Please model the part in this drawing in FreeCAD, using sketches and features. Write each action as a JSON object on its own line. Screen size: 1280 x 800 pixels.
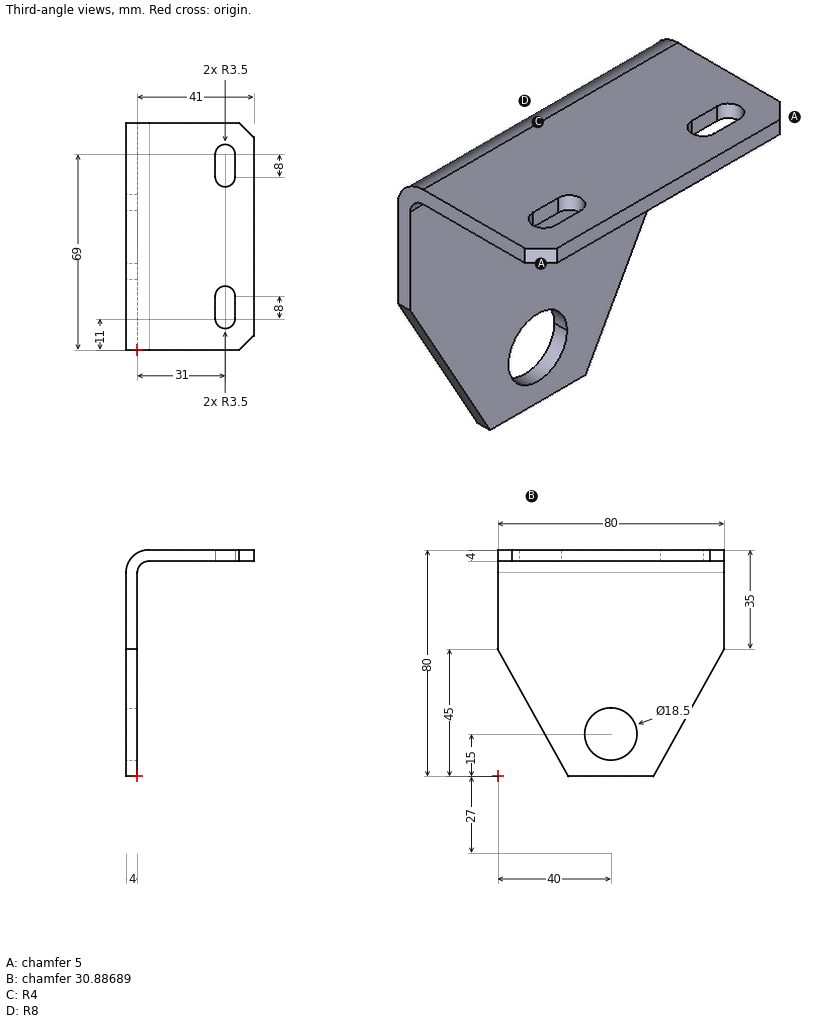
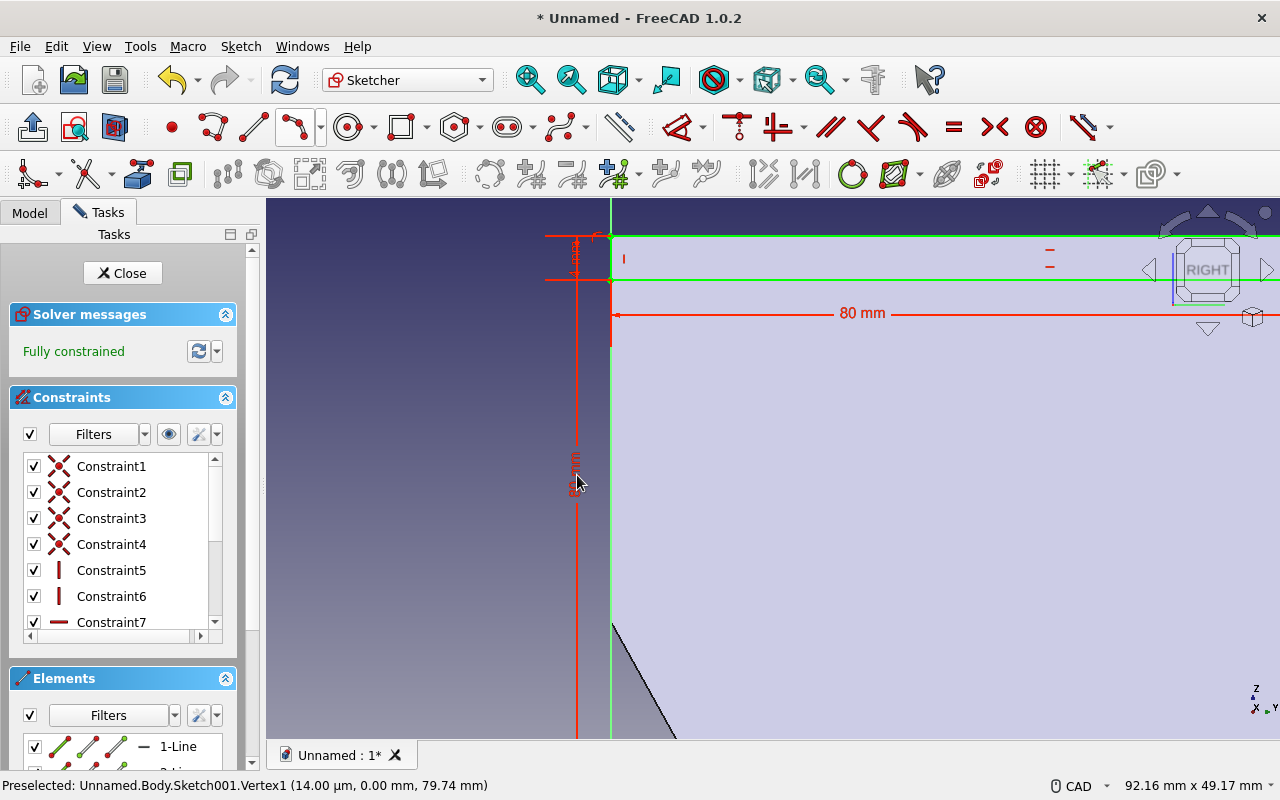
{"action": "left_click", "coordinate": [123, 273]}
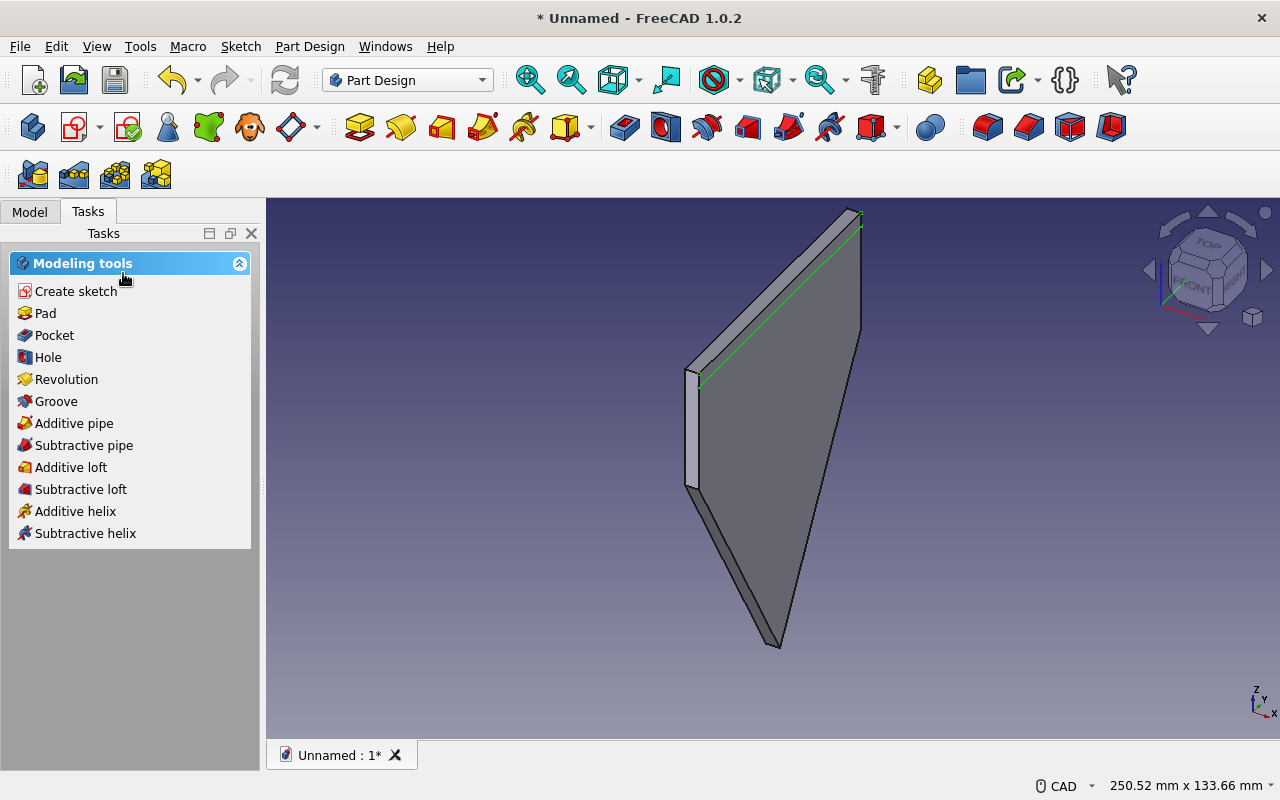
{"action": "left_click", "coordinate": [360, 128]}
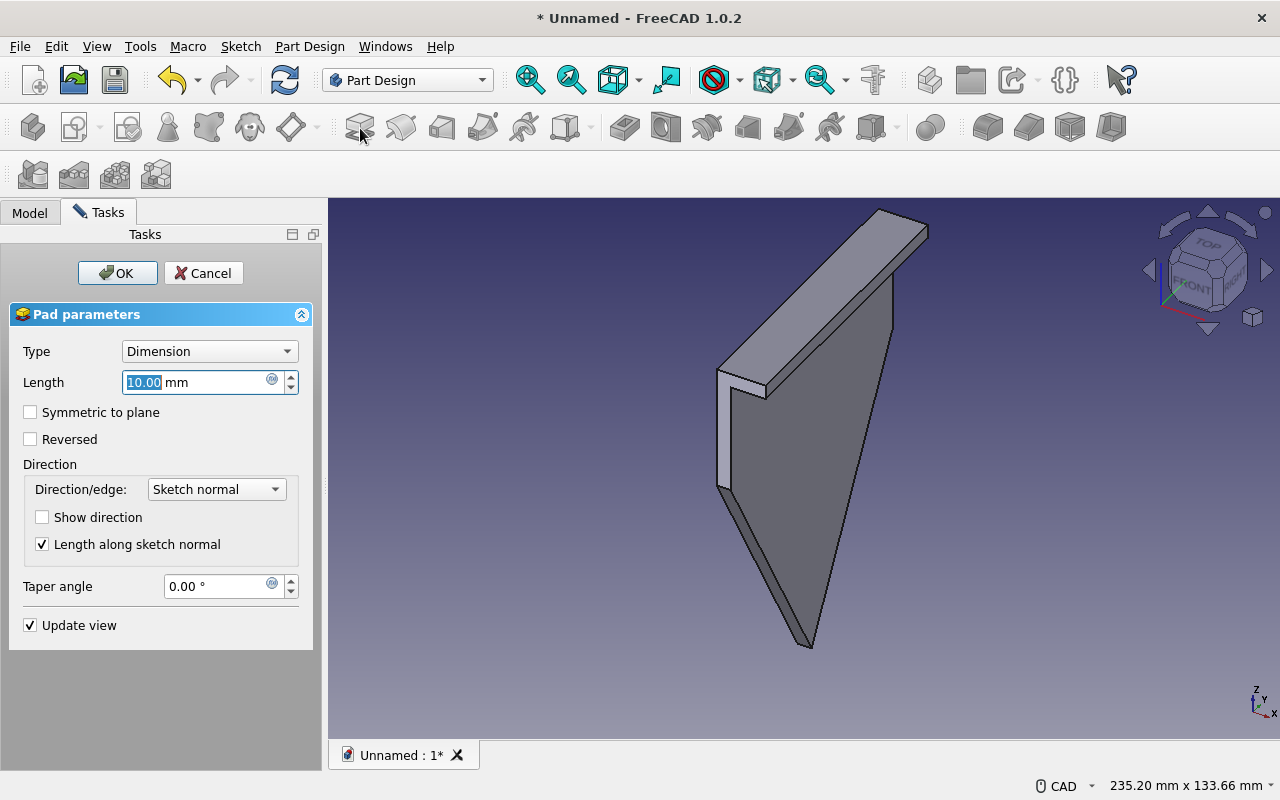
{"action": "type", "text": "41"}
{"action": "key", "text": "Tab"}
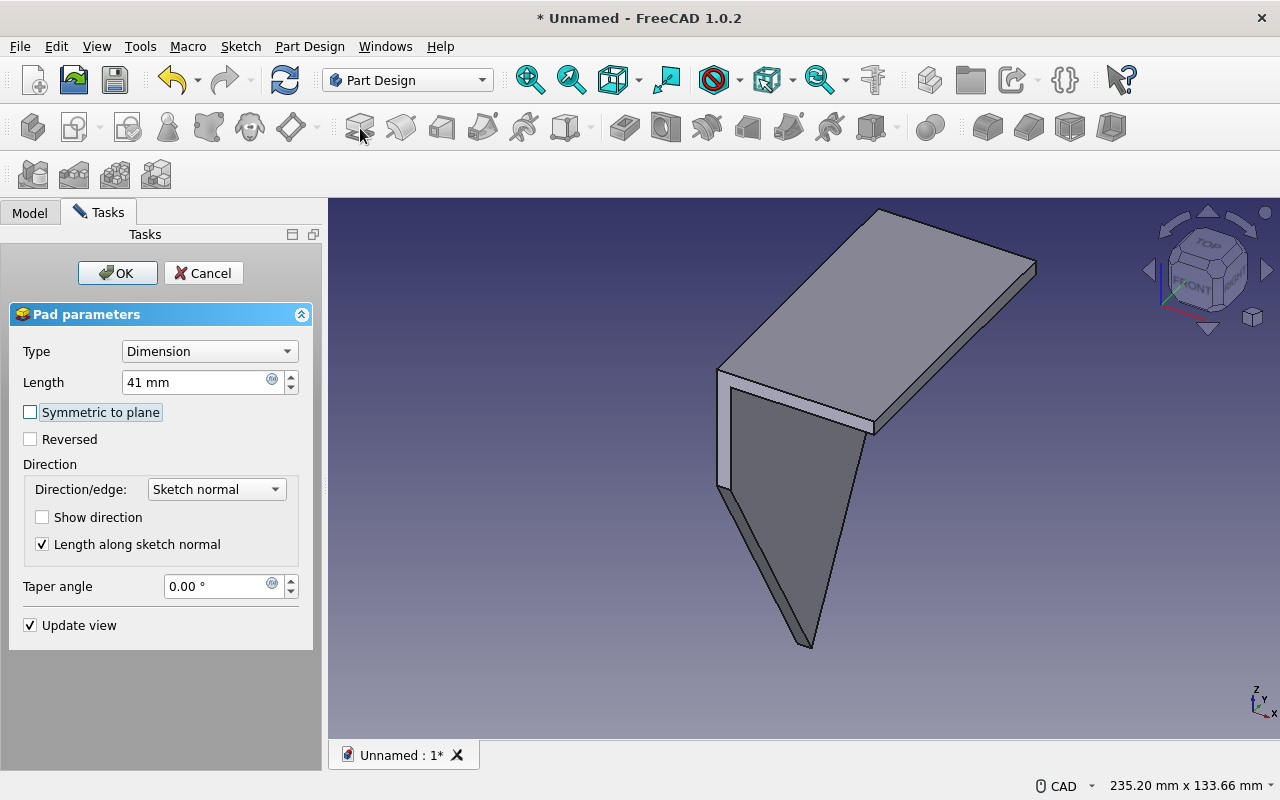
{"action": "left_click", "coordinate": [118, 273]}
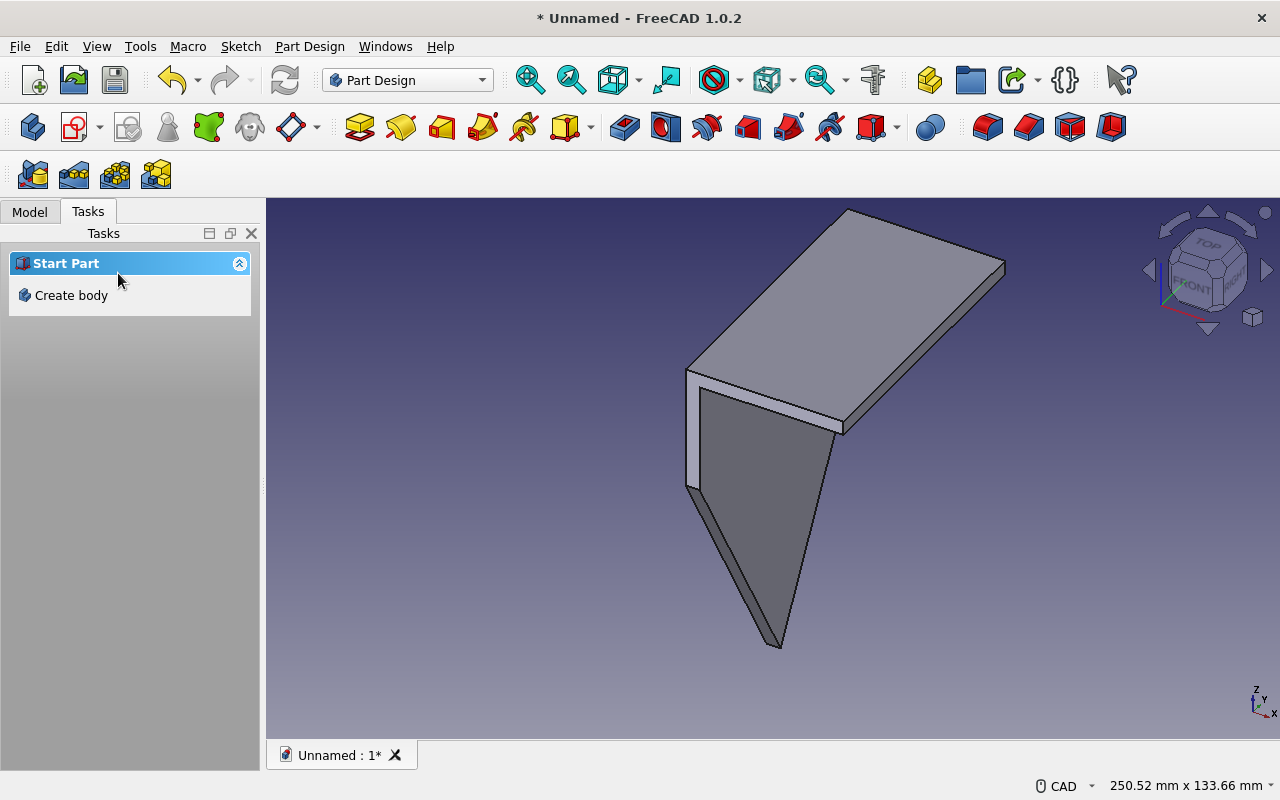
{"action": "key", "text": "v f"}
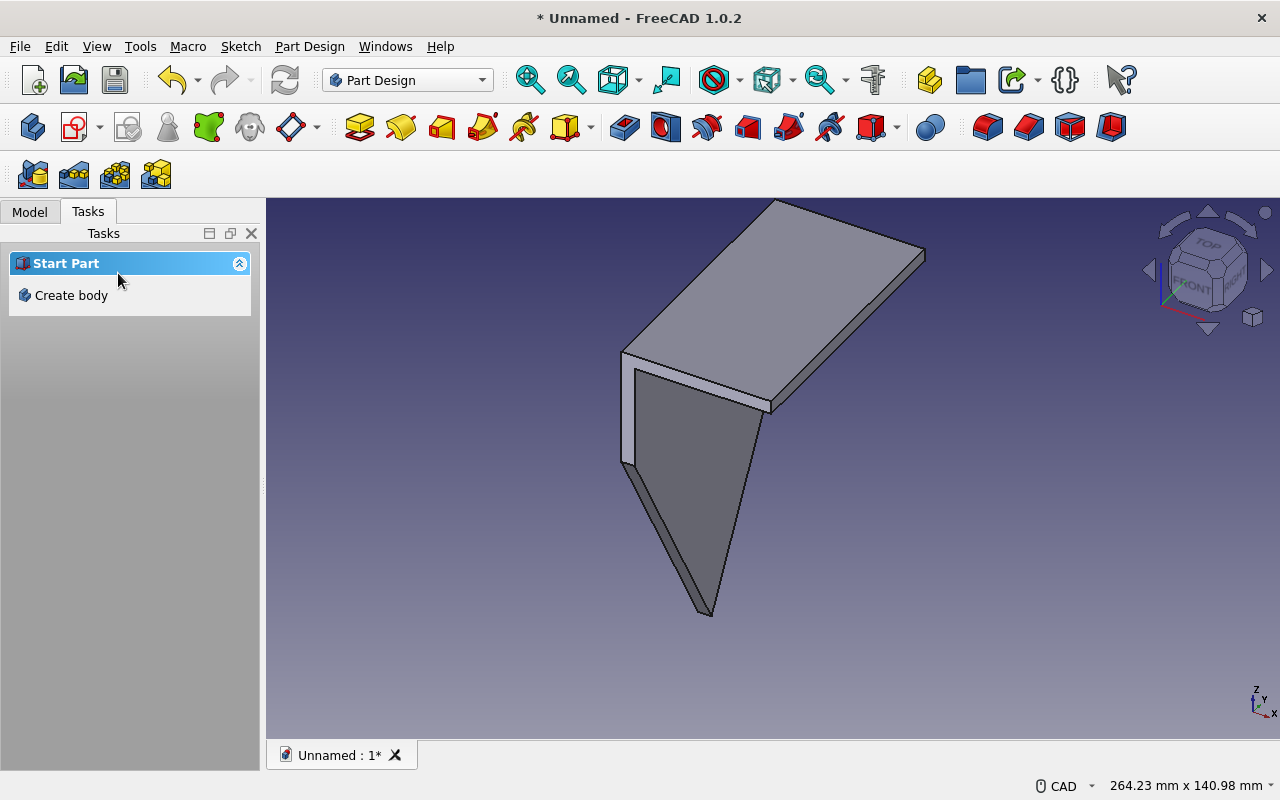
{"action": "left_click", "coordinate": [795, 278]}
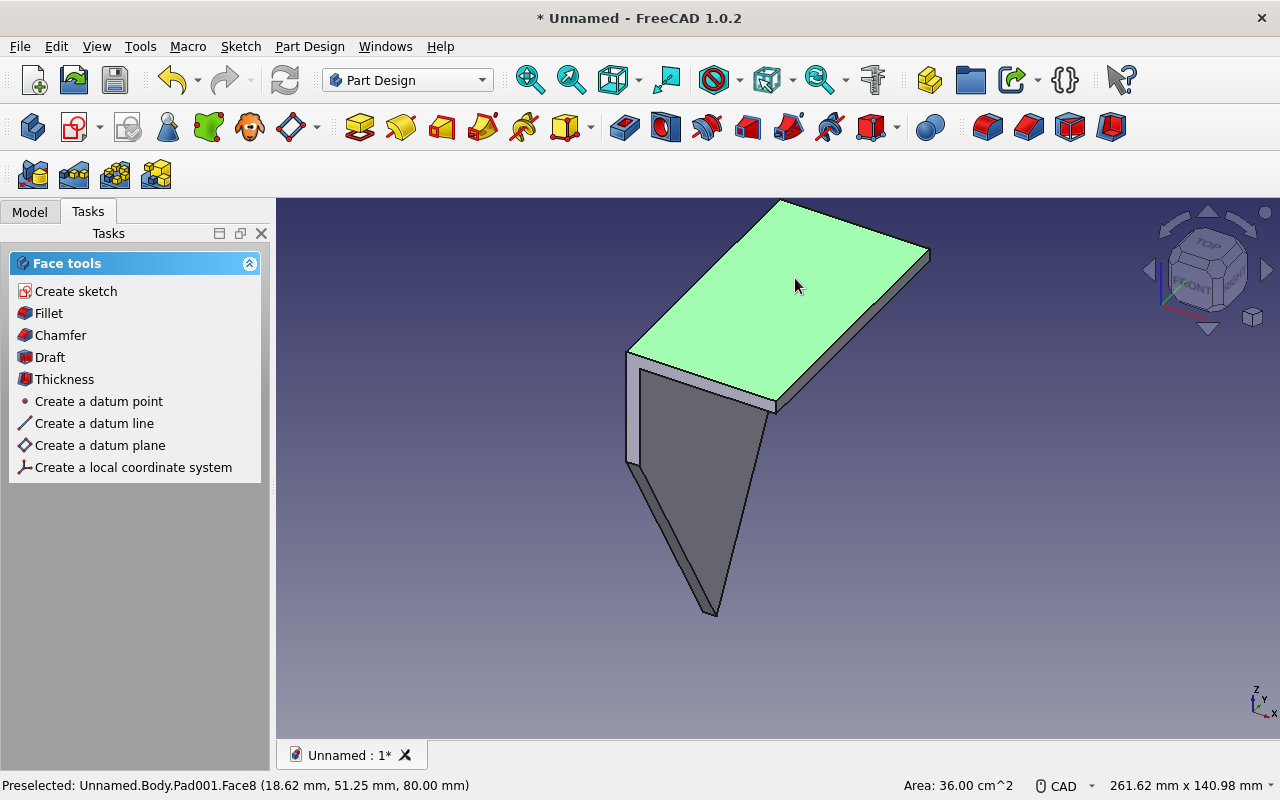
{"action": "left_click", "coordinate": [74, 128]}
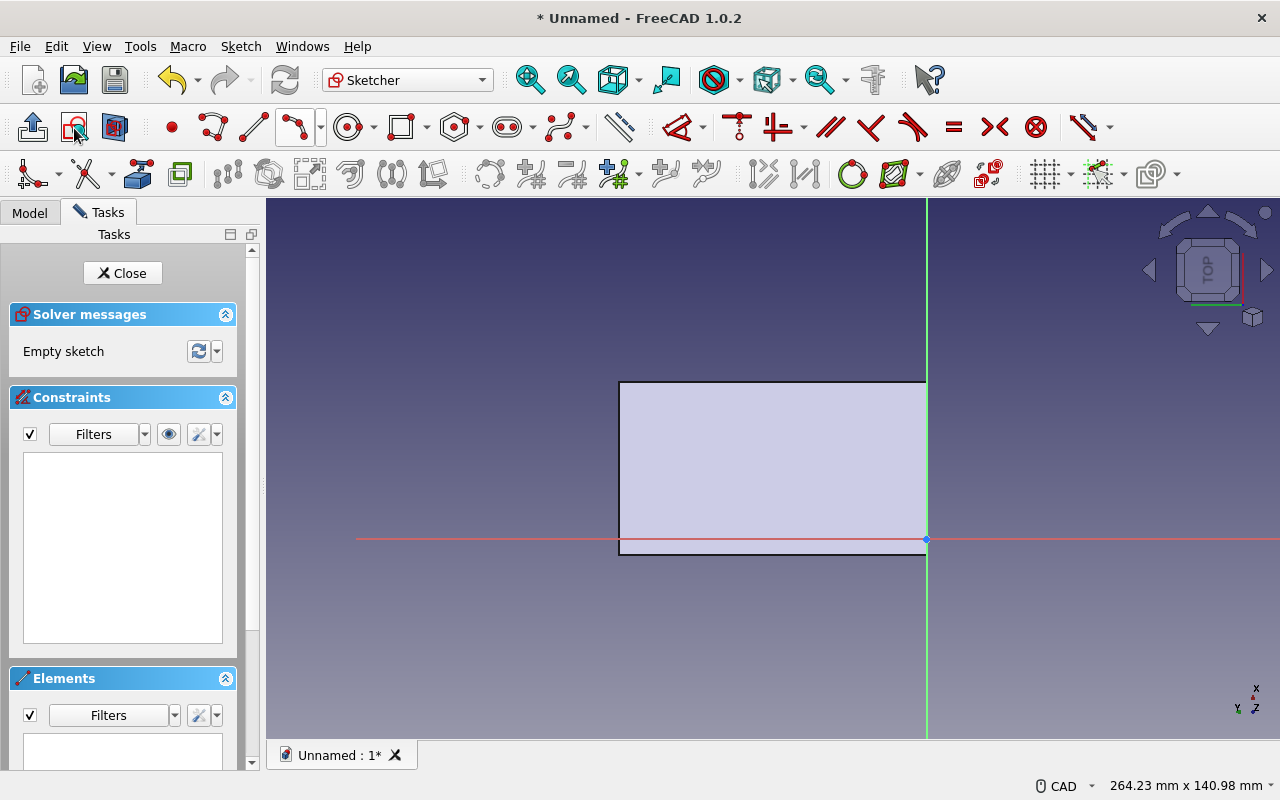
{"action": "scroll", "coordinate": [674, 416], "scroll_direction": "up", "scroll_amount": 12}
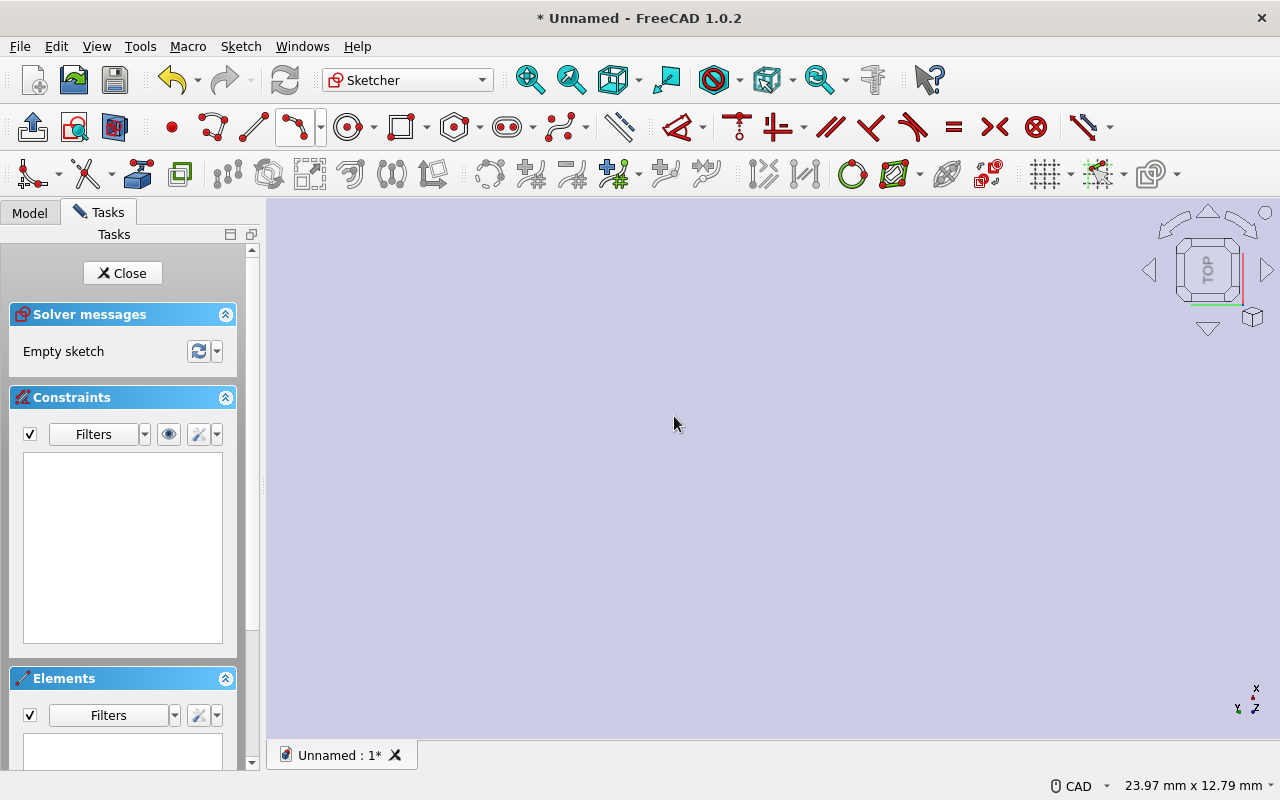
{"action": "key", "text": "g s"}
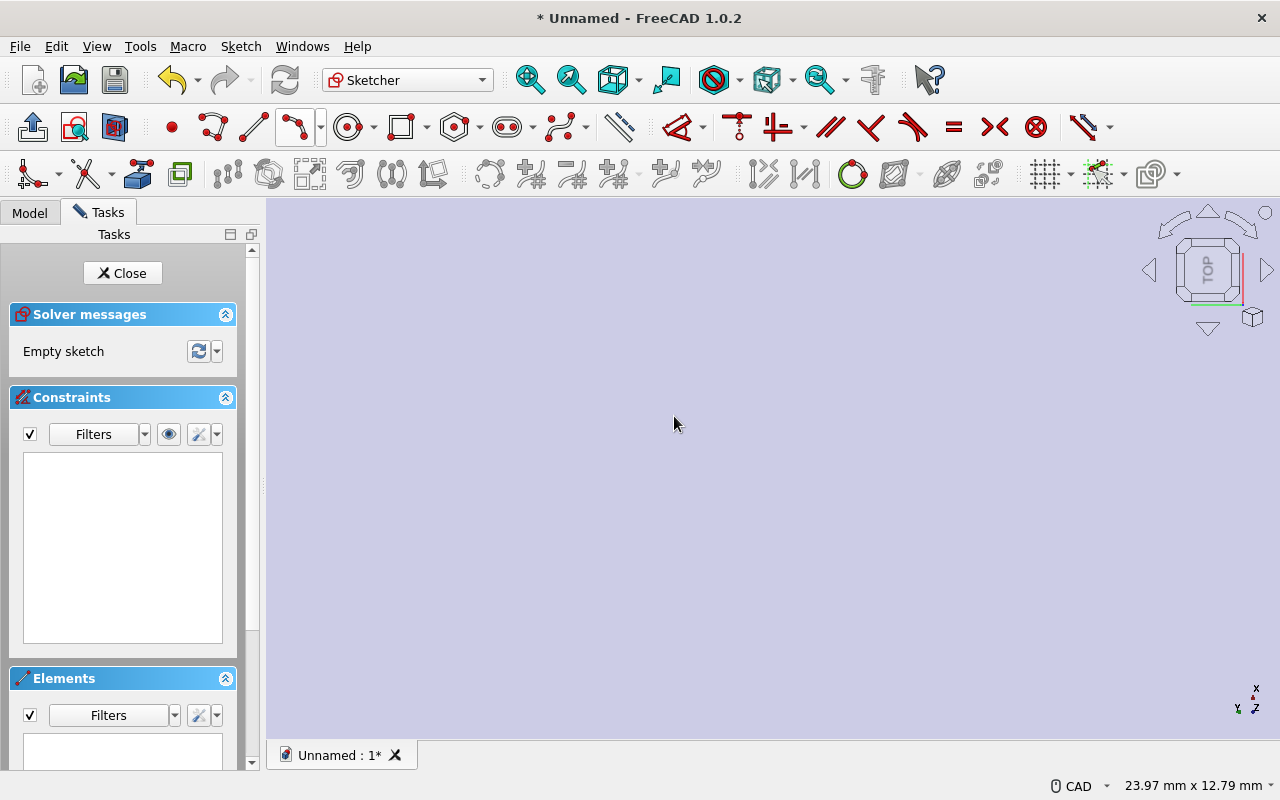
{"action": "left_click", "coordinate": [534, 462]}